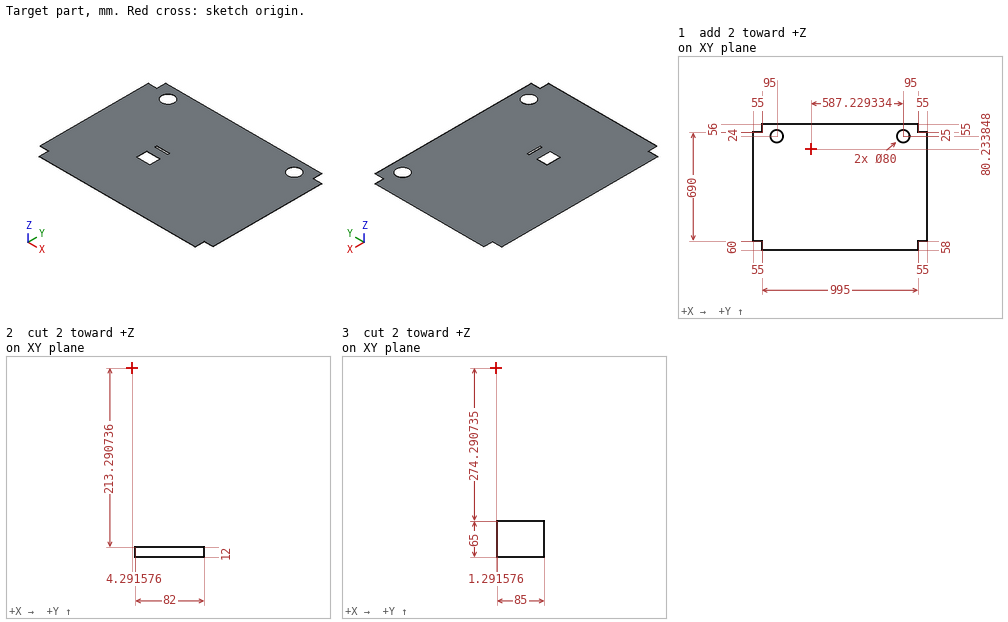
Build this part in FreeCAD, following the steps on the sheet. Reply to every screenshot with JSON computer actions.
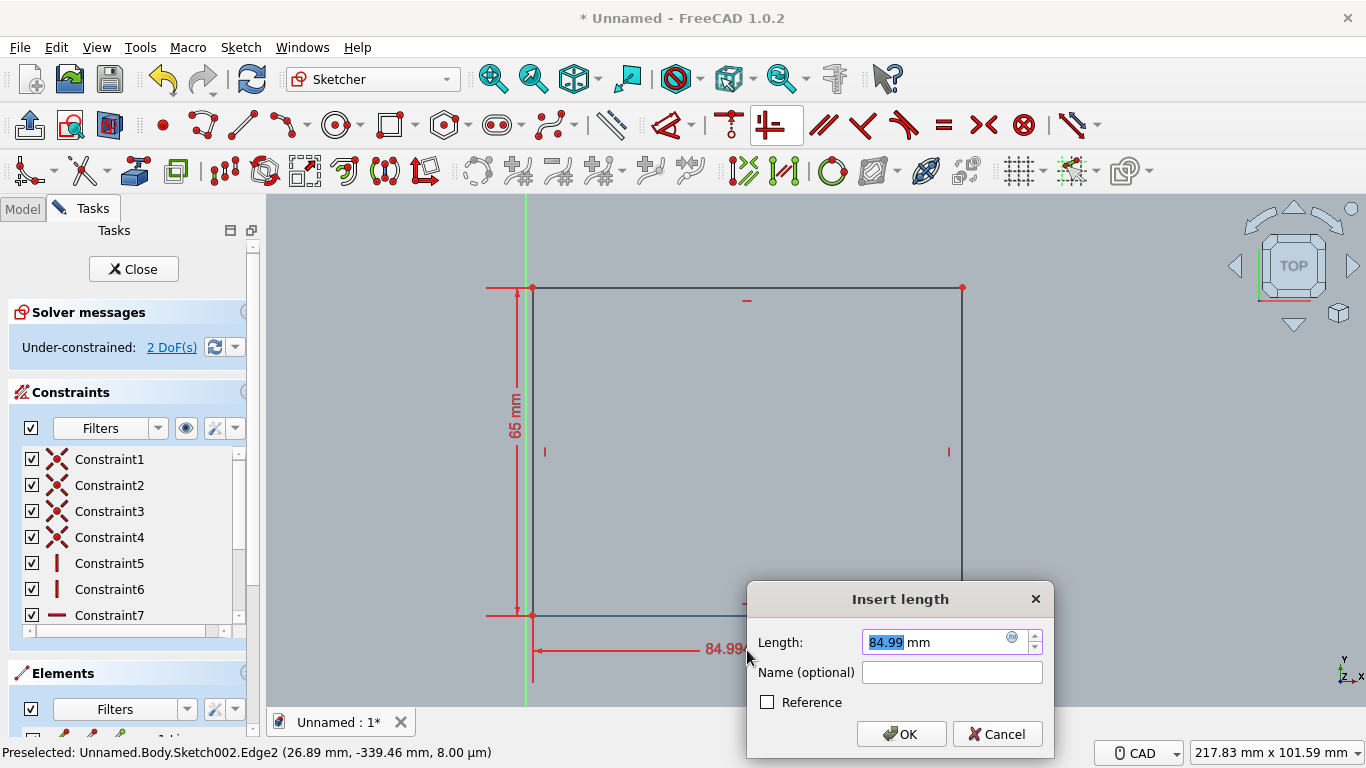
{"action": "type", "text": "85"}
{"action": "key", "text": "Return"}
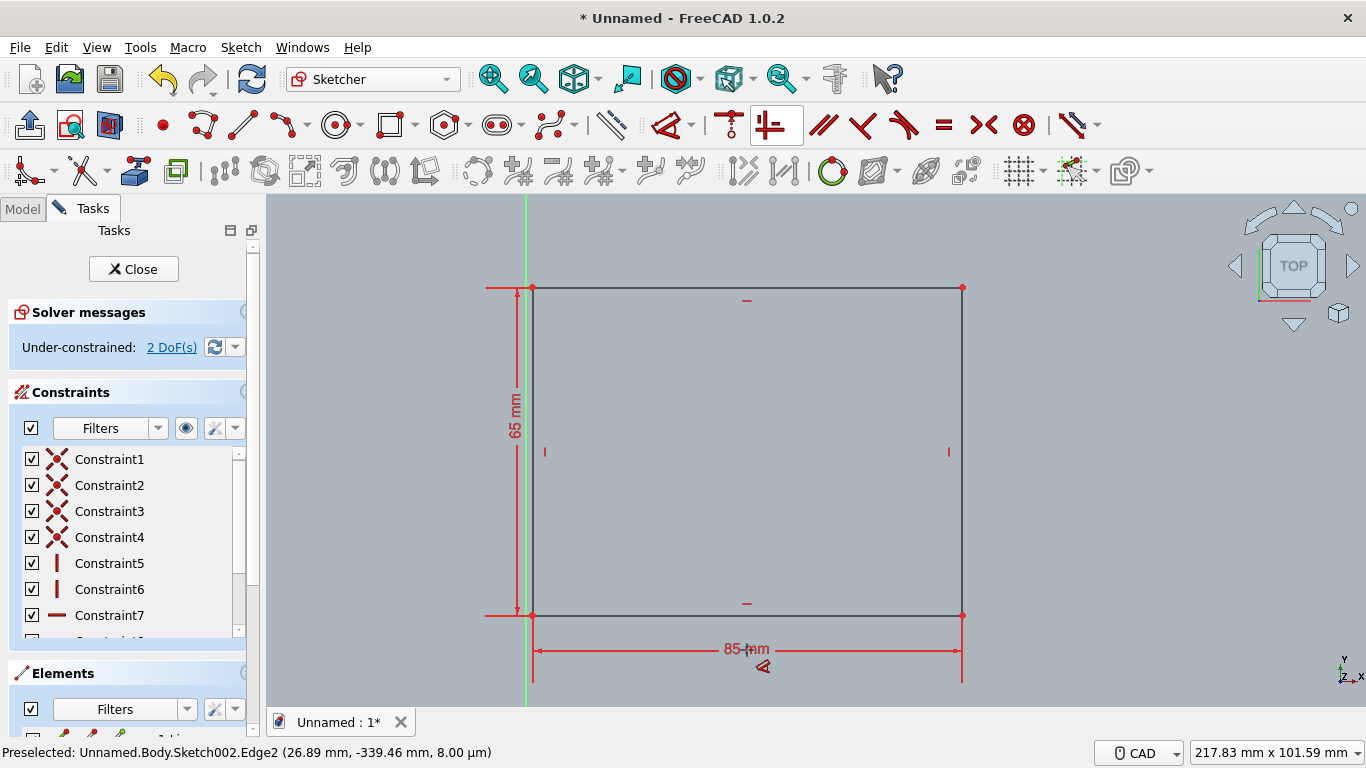
{"action": "scroll", "coordinate": [533, 288], "scroll_direction": "up", "scroll_amount": 10}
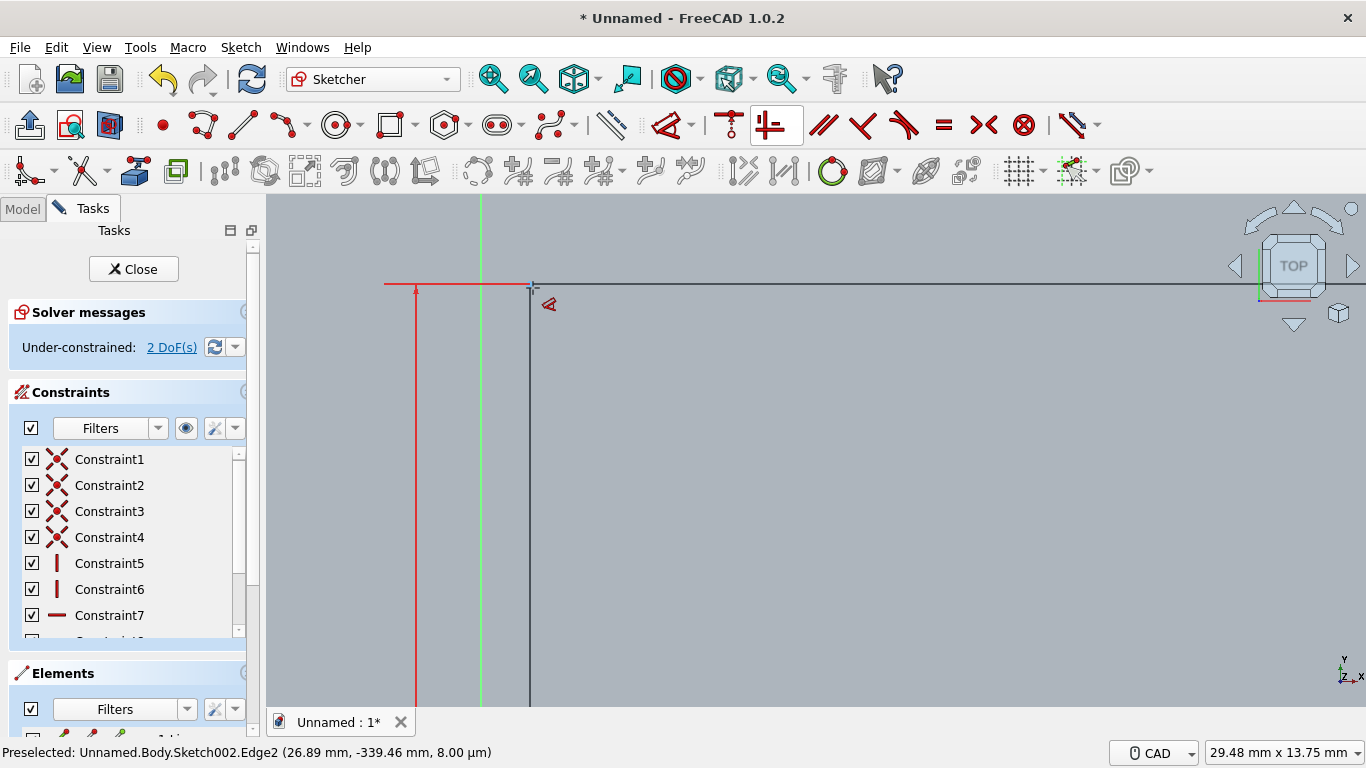
{"action": "left_click", "coordinate": [530, 284]}
{"action": "left_click", "coordinate": [506, 318]}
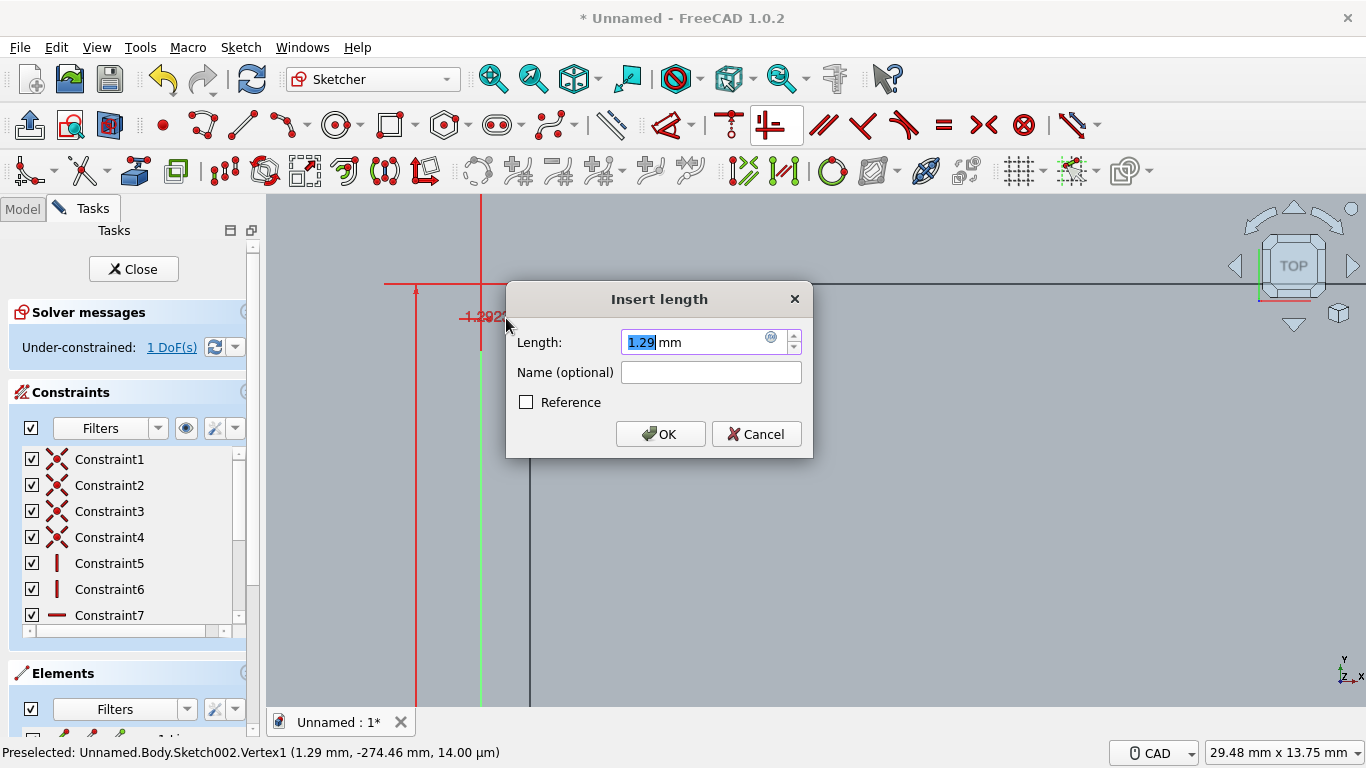
{"action": "type", "text": "1.291576"}
{"action": "key", "text": "Return"}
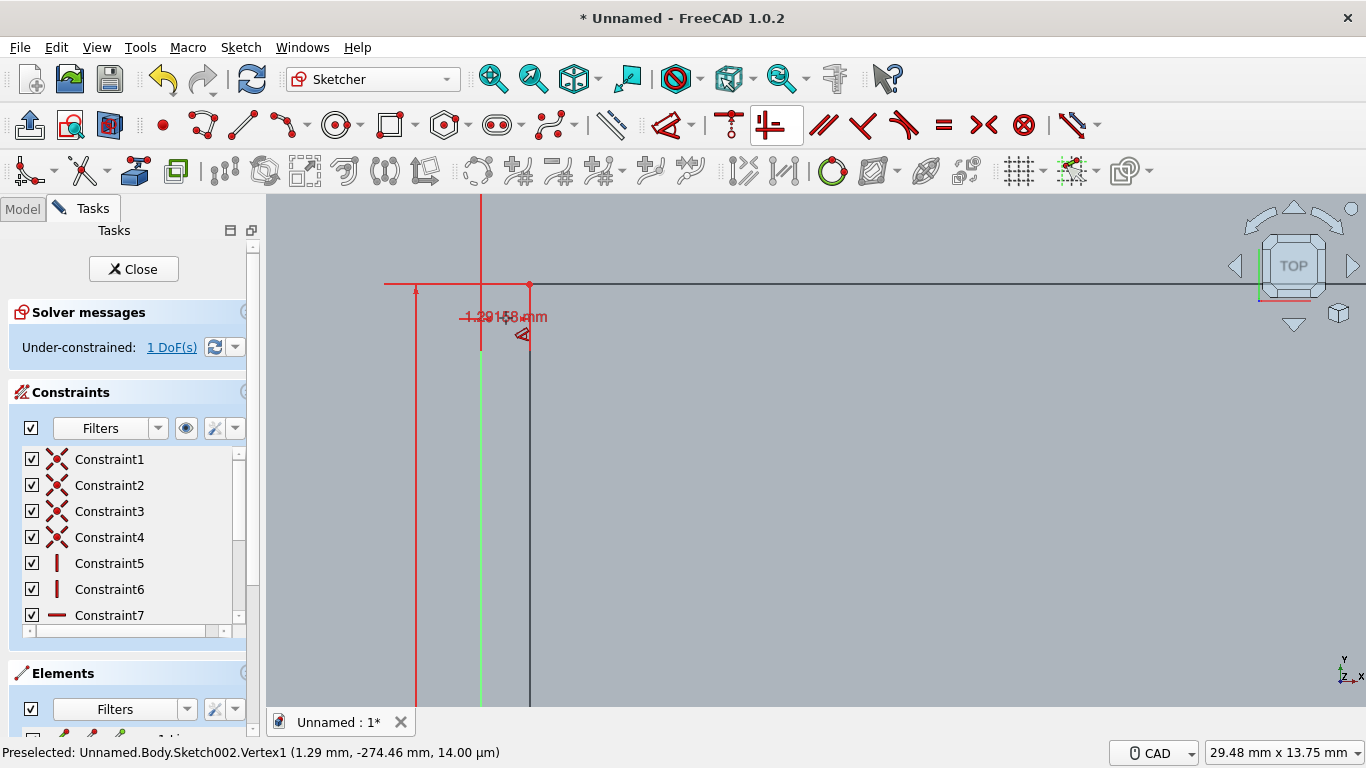
{"action": "scroll", "coordinate": [533, 288], "scroll_direction": "down", "scroll_amount": 10}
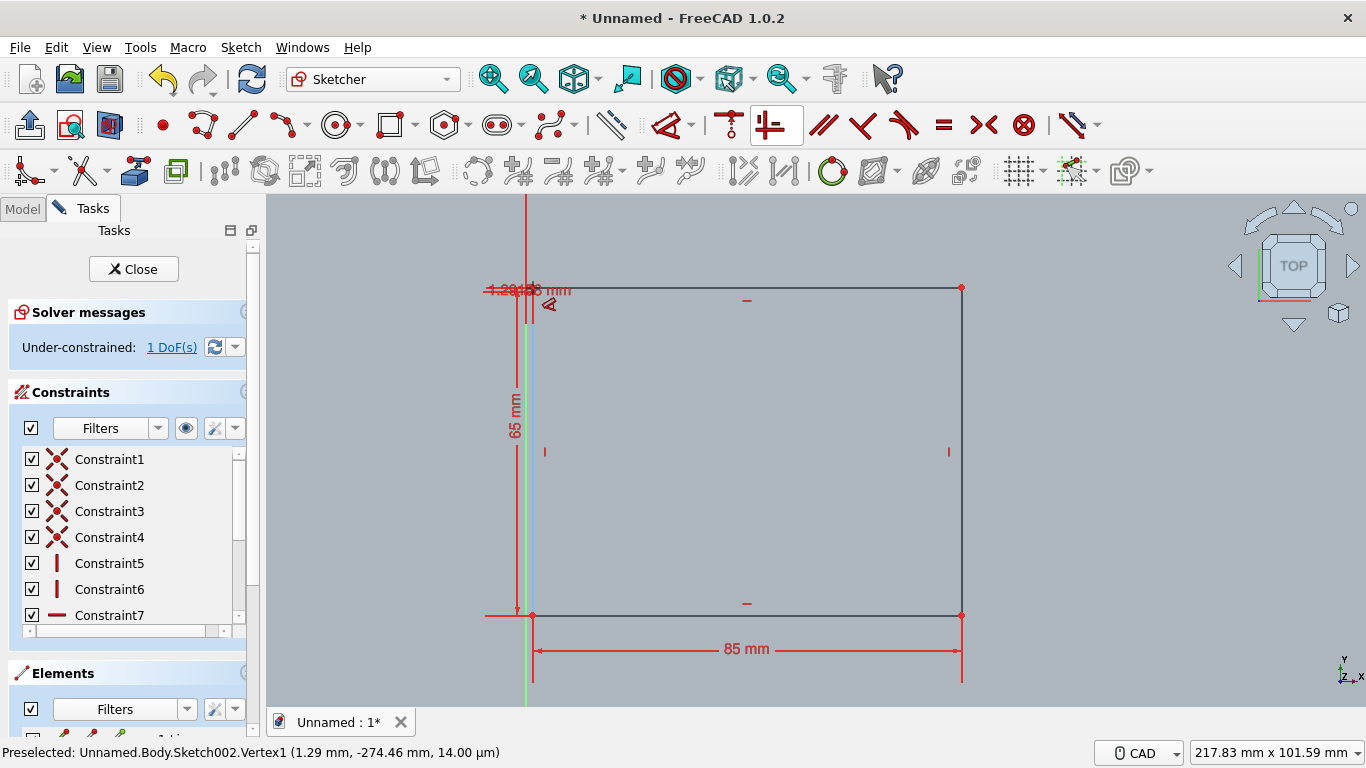
{"action": "left_click", "coordinate": [533, 288]}
{"action": "left_click", "coordinate": [492, 255]}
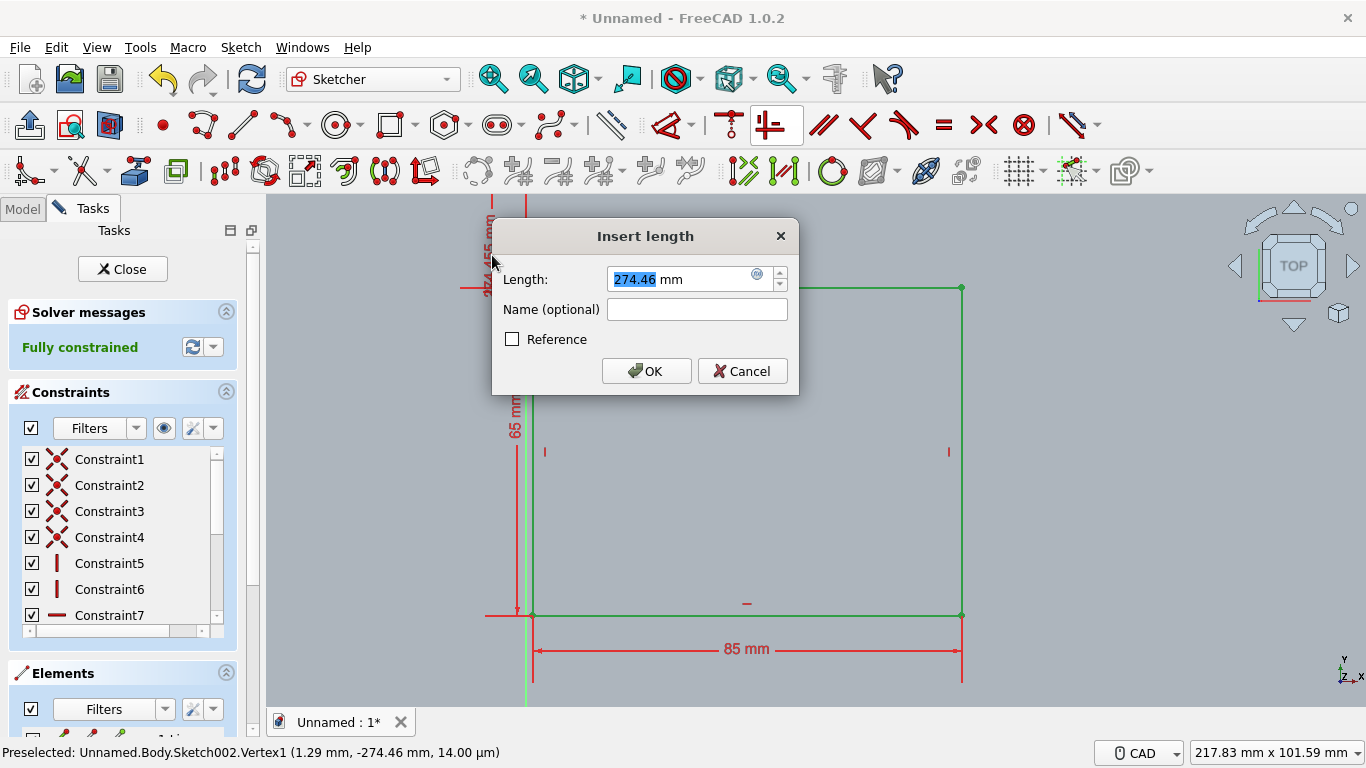
{"action": "type", "text": "274.290735"}
{"action": "key", "text": "Return"}
{"action": "key", "text": "Escape"}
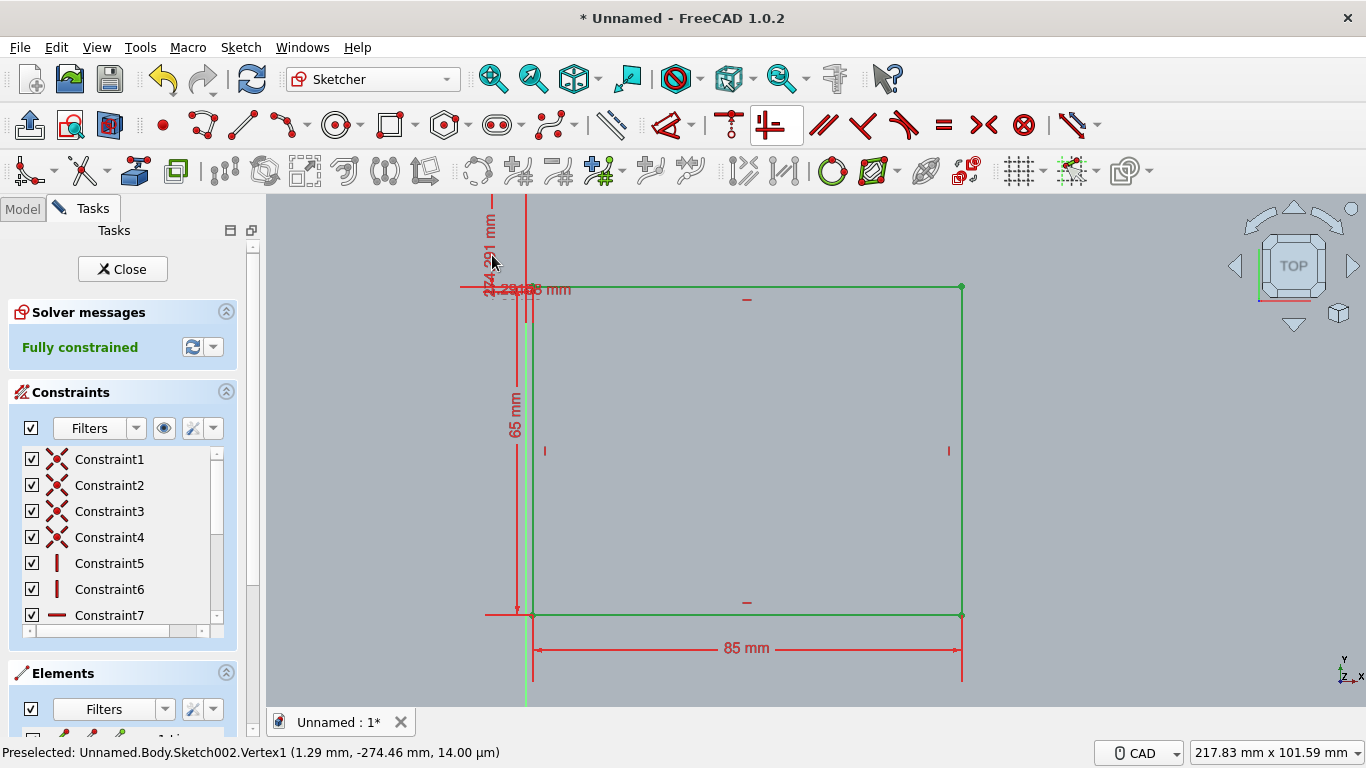
{"action": "left_click", "coordinate": [123, 269]}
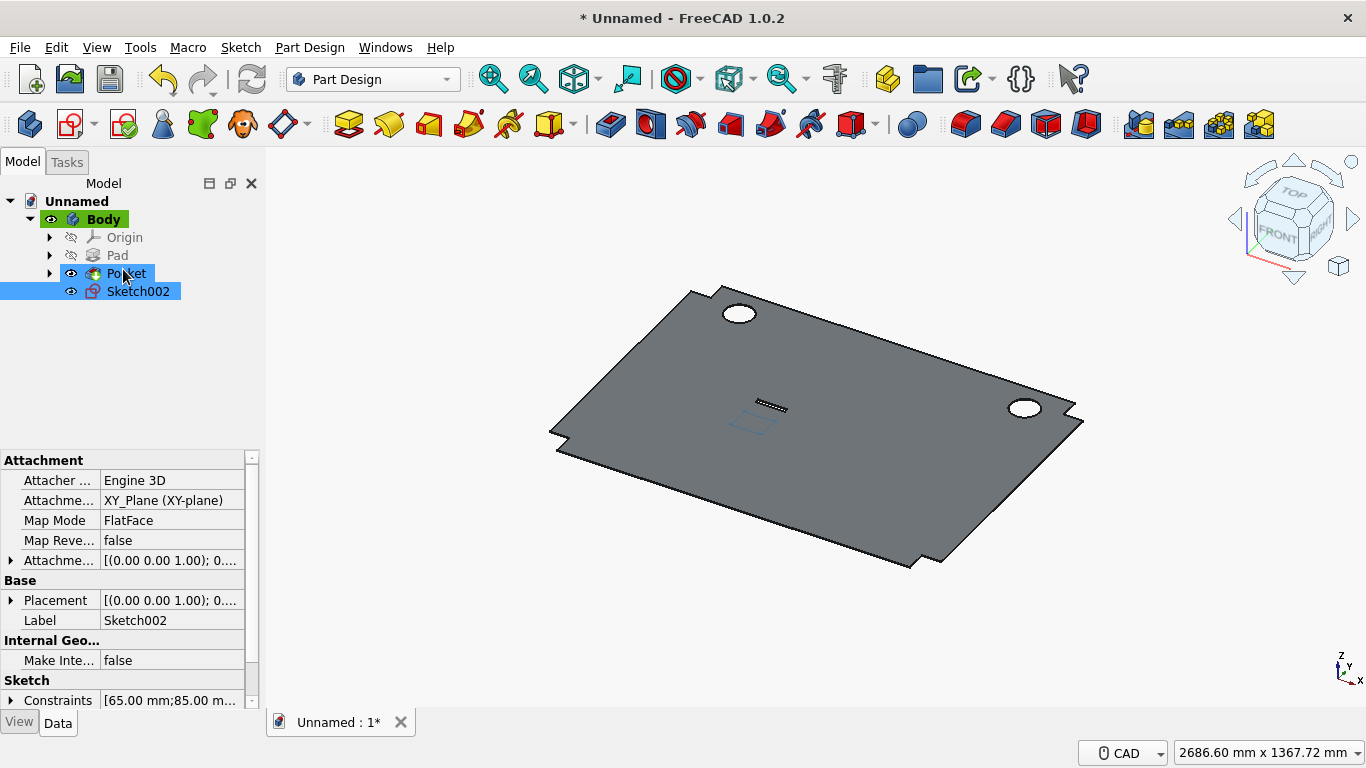
{"action": "left_click", "coordinate": [612, 124]}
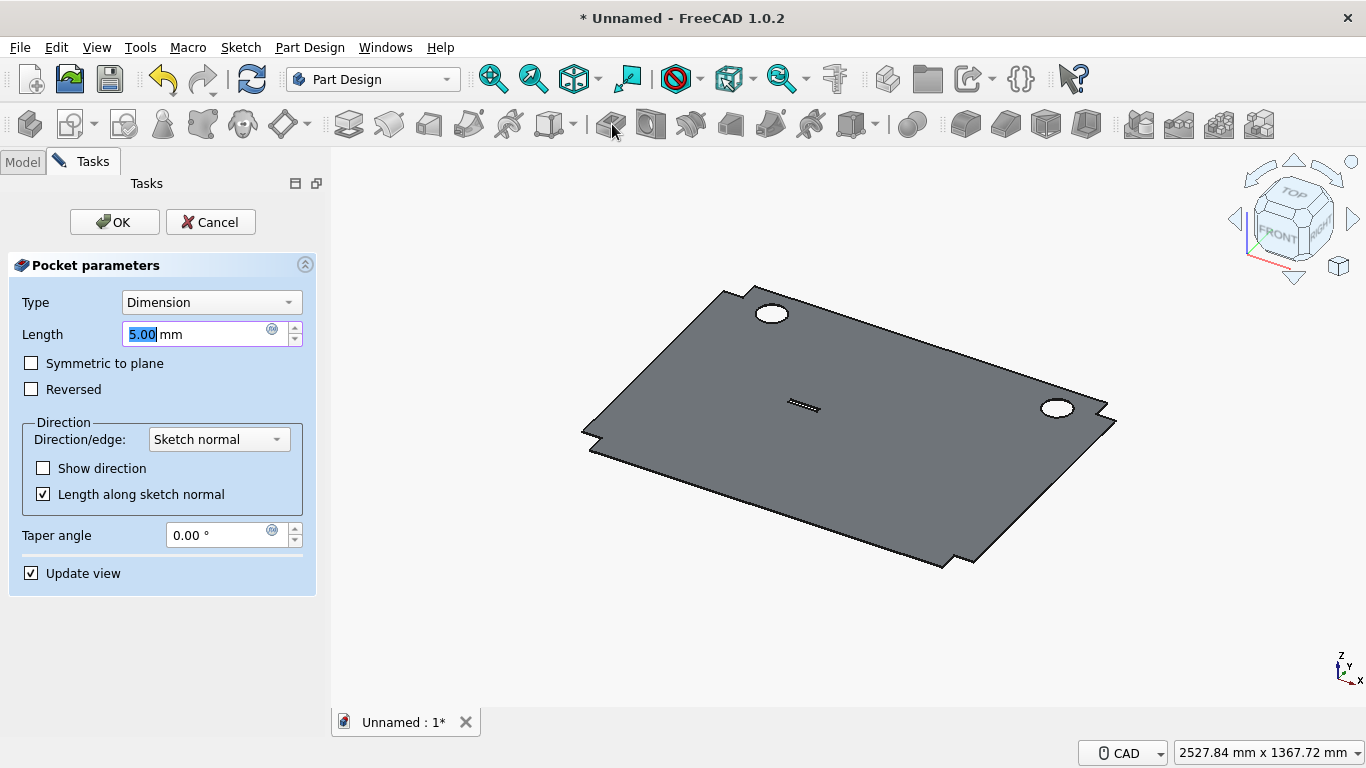
{"action": "type", "text": "2"}
{"action": "key", "text": "Tab"}